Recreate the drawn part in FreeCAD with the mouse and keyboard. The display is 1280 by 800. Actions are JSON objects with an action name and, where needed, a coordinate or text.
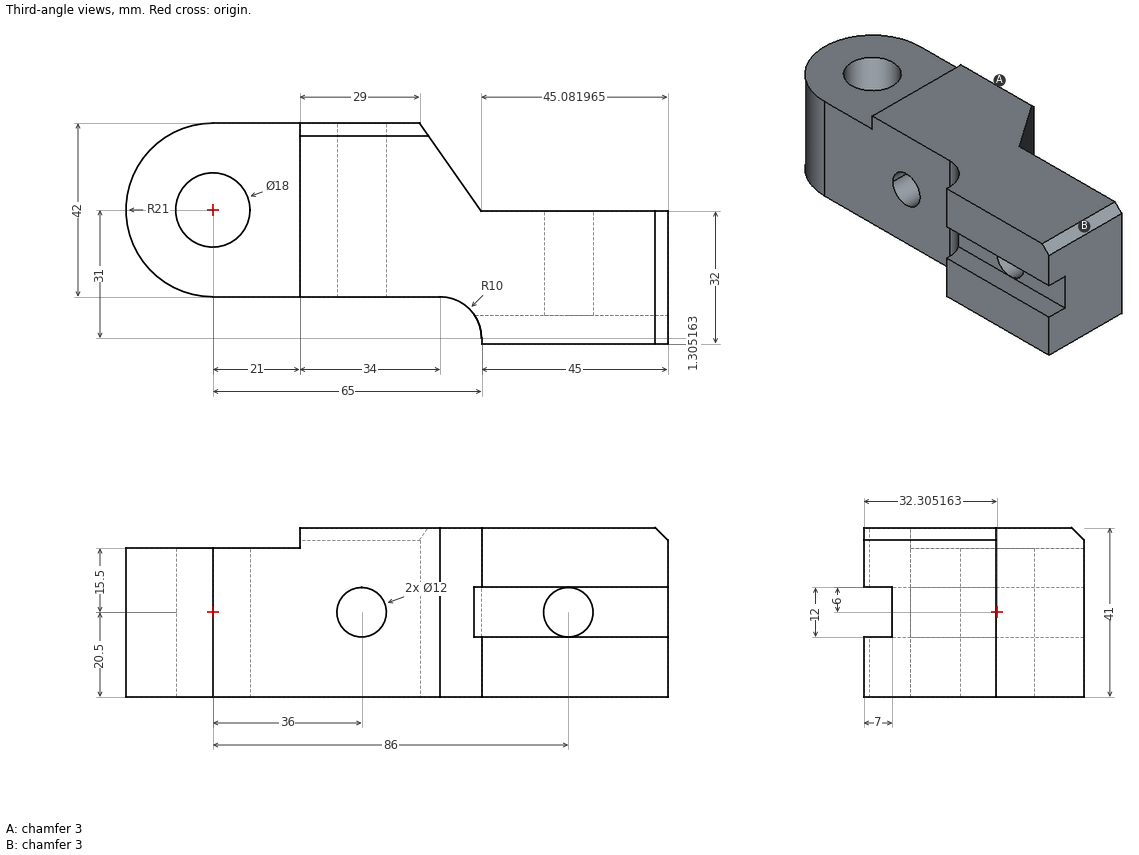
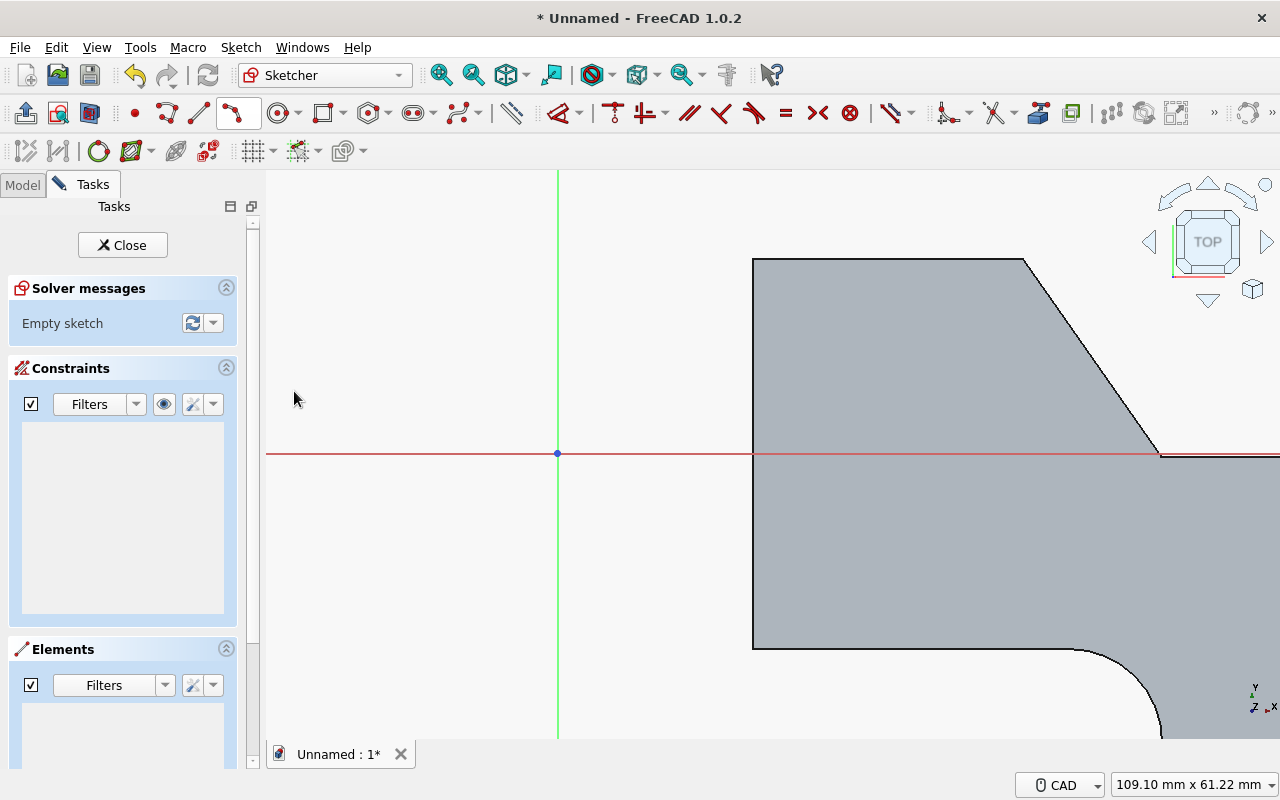
{"action": "left_click", "coordinate": [168, 114]}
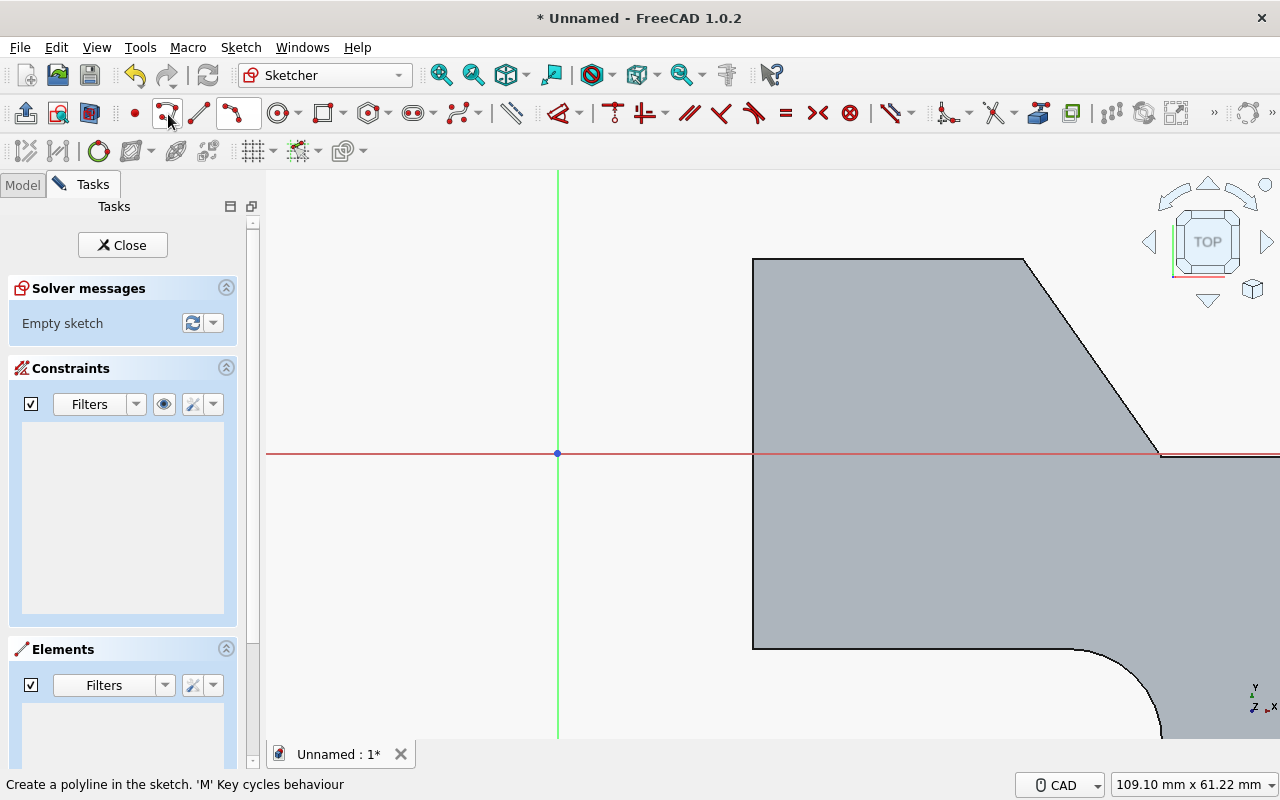
{"action": "left_click", "coordinate": [558, 649]}
{"action": "left_click", "coordinate": [753, 649]}
{"action": "left_click", "coordinate": [753, 259]}
{"action": "left_click", "coordinate": [558, 259]}
{"action": "right_click", "coordinate": [558, 259]}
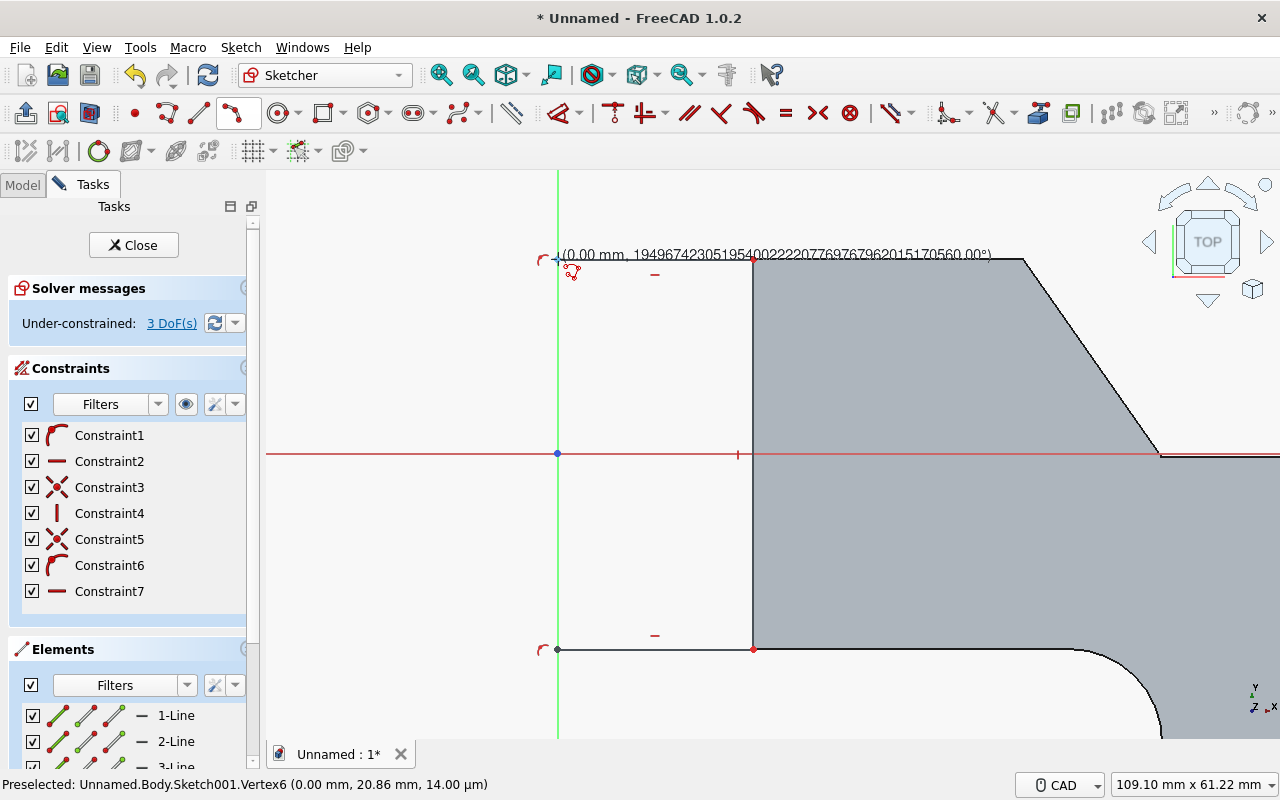
{"action": "left_click", "coordinate": [232, 114]}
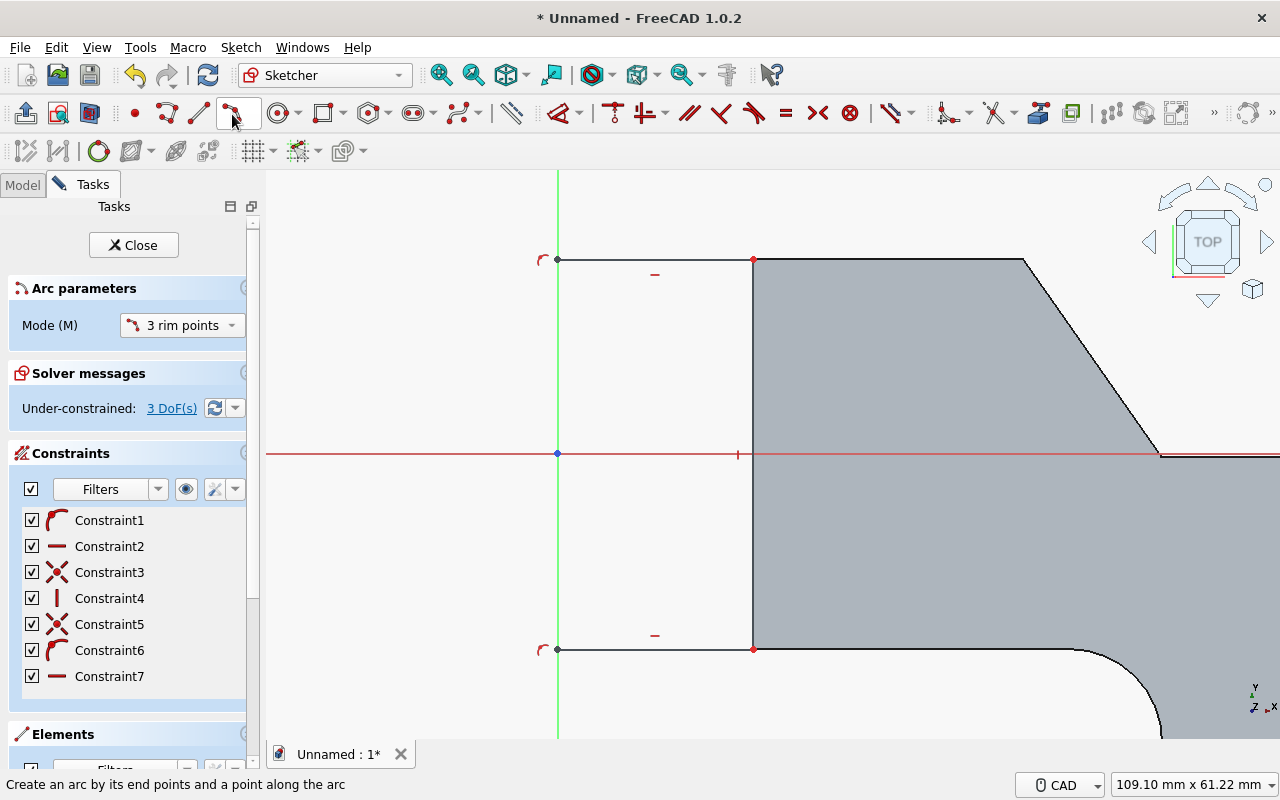
{"action": "left_click", "coordinate": [558, 260]}
{"action": "left_click", "coordinate": [558, 650]}
{"action": "left_click", "coordinate": [372, 394]}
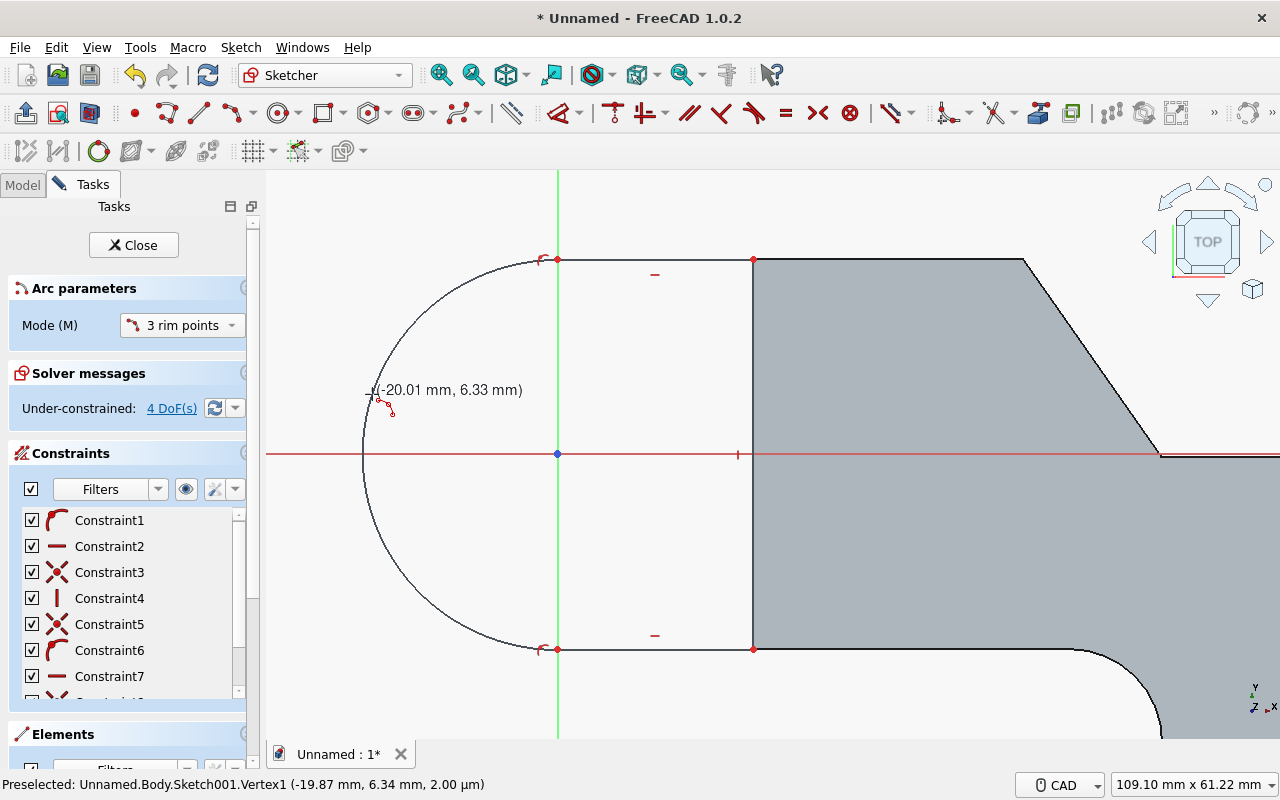
{"action": "left_click", "coordinate": [278, 114]}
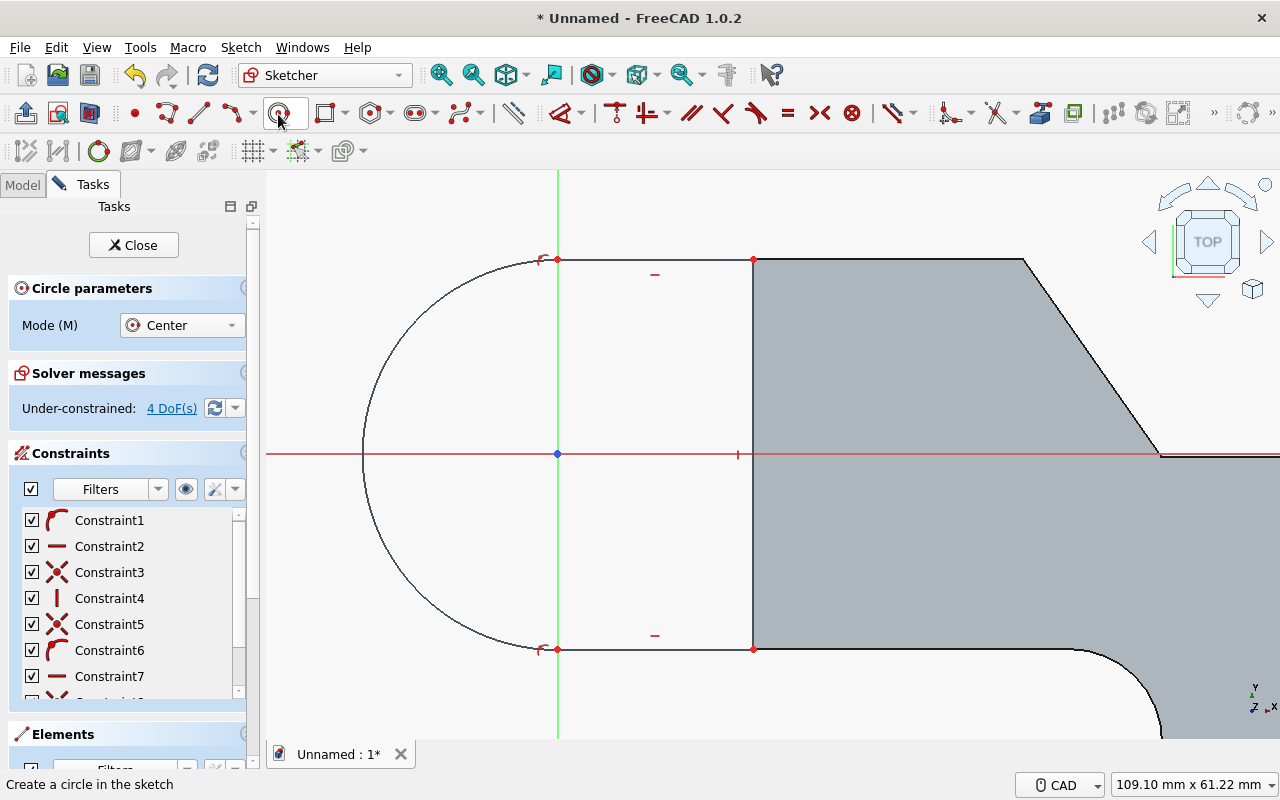
{"action": "left_click", "coordinate": [558, 454]}
{"action": "mouse_move", "coordinate": [617, 395]}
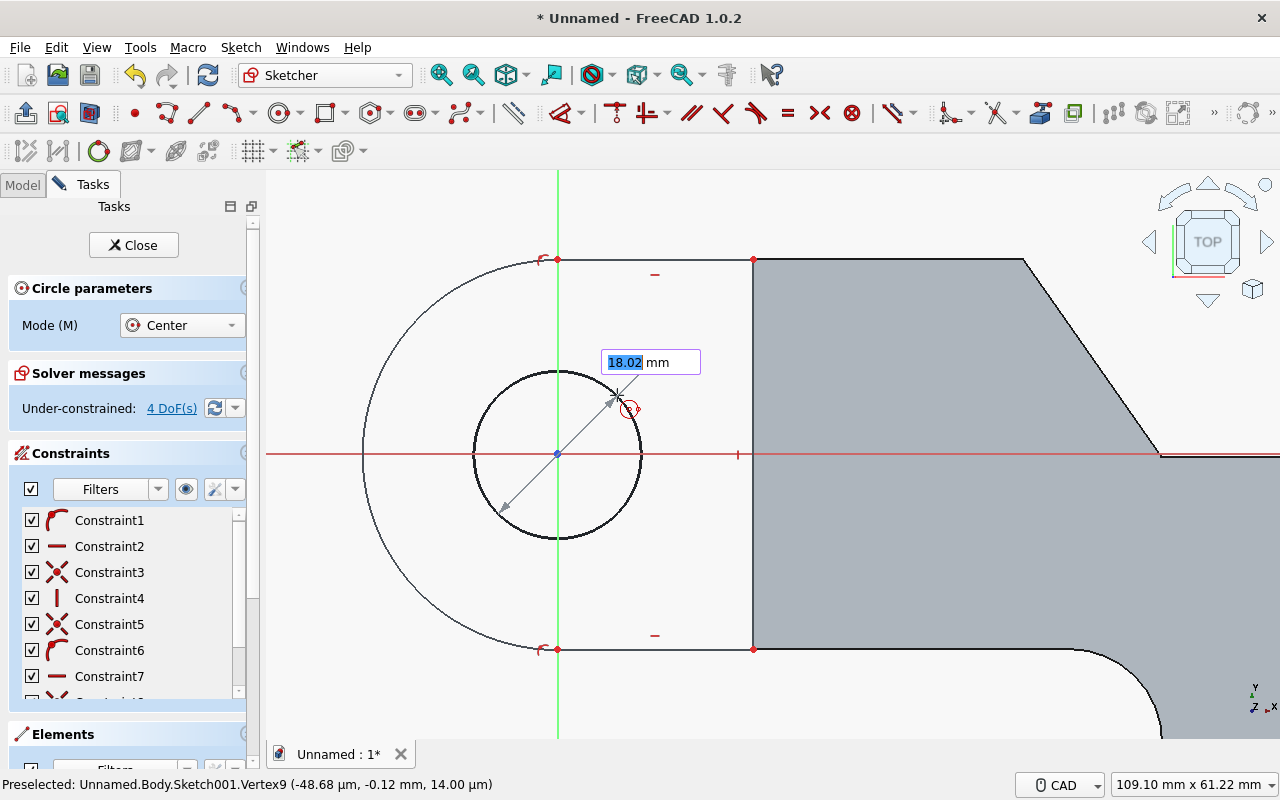
{"action": "type", "text": "18"}
{"action": "key", "text": "Return"}
{"action": "key", "text": "Escape"}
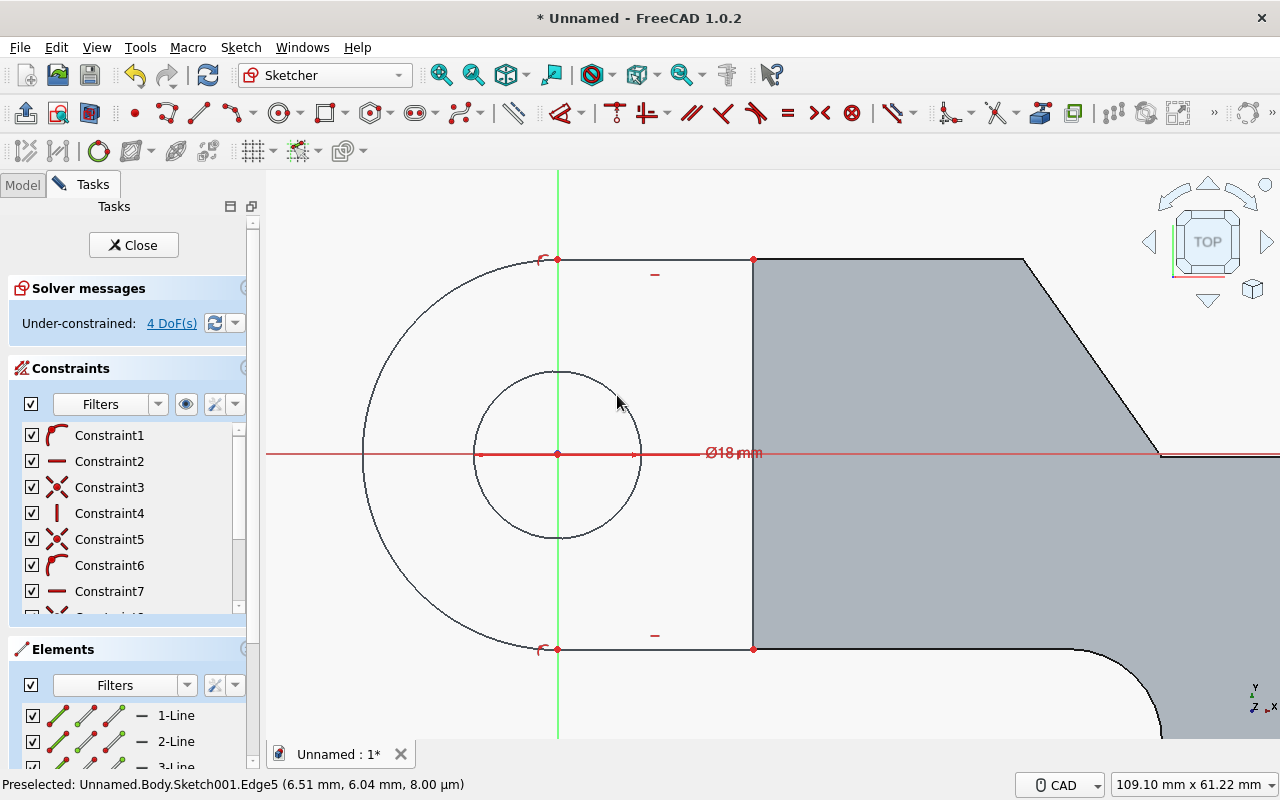
{"action": "left_click", "coordinate": [616, 650]}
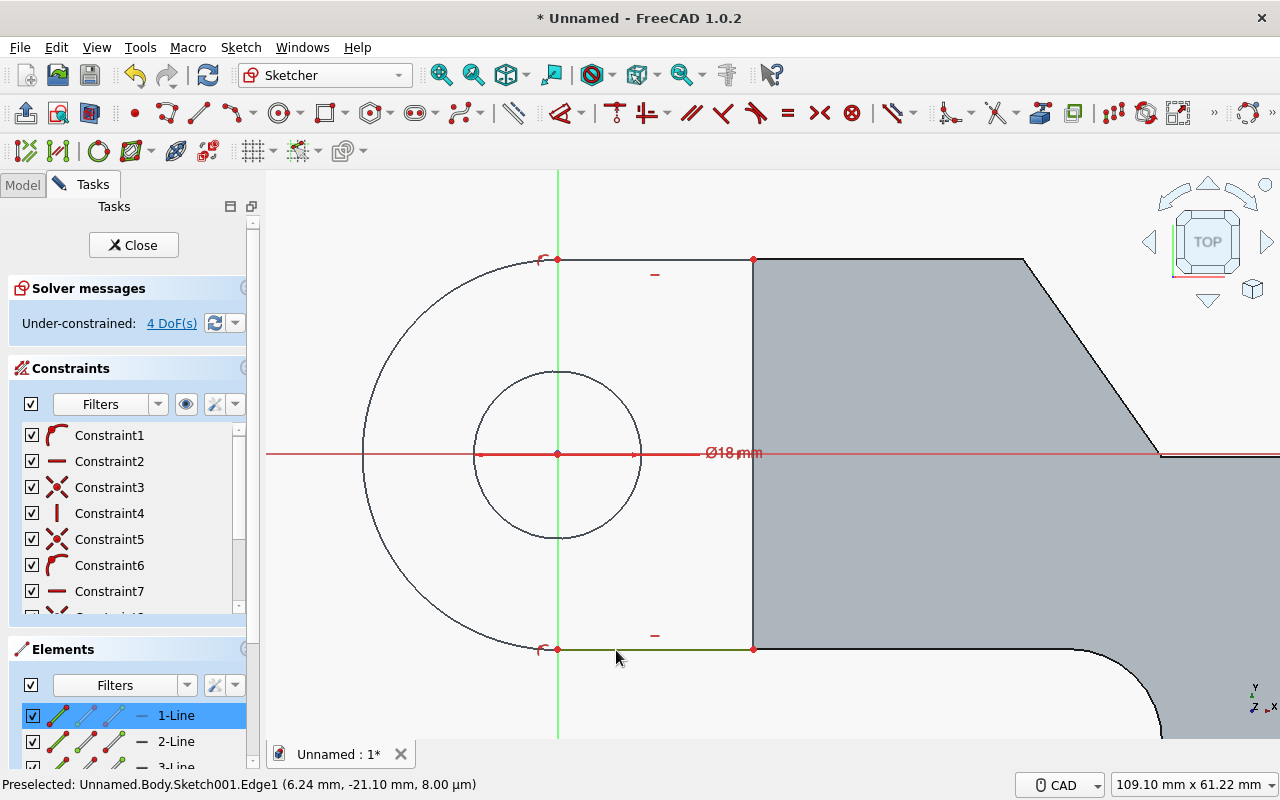
{"action": "left_click", "coordinate": [400, 340]}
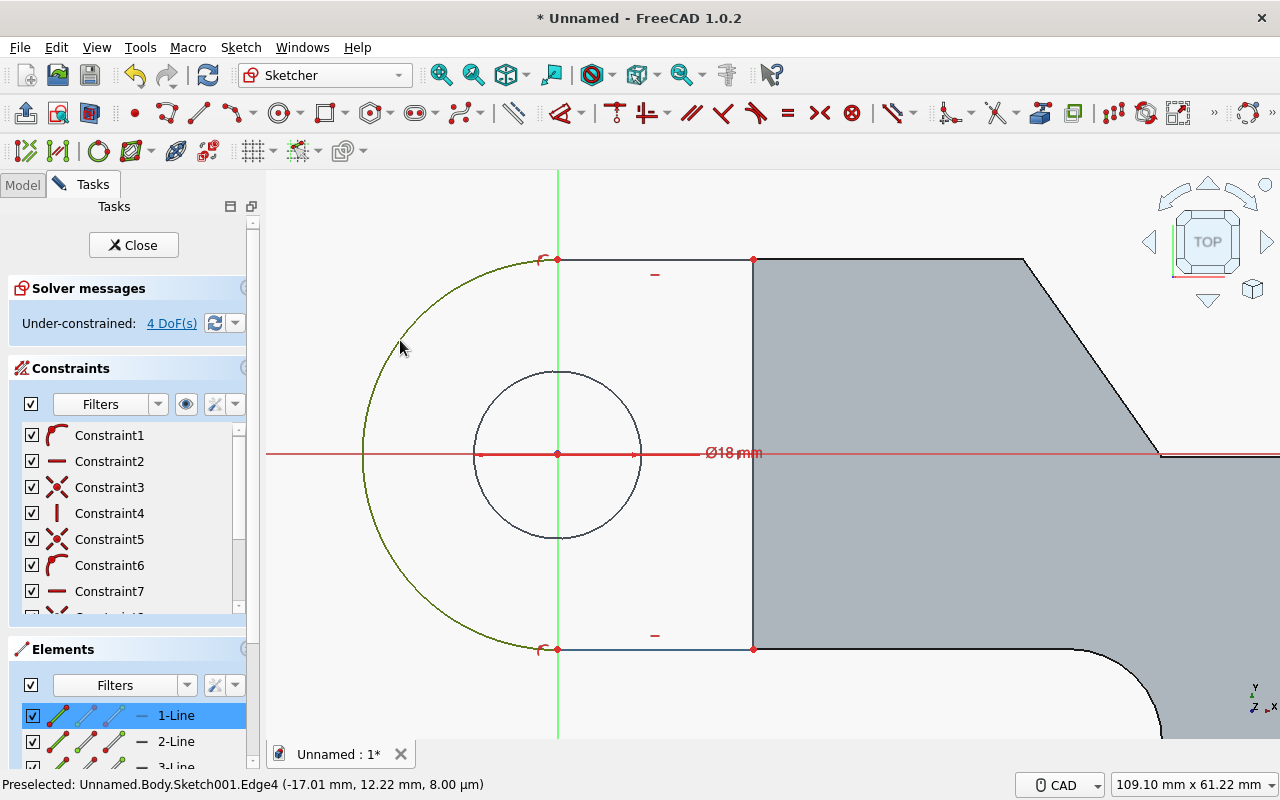
{"action": "left_click", "coordinate": [756, 114]}